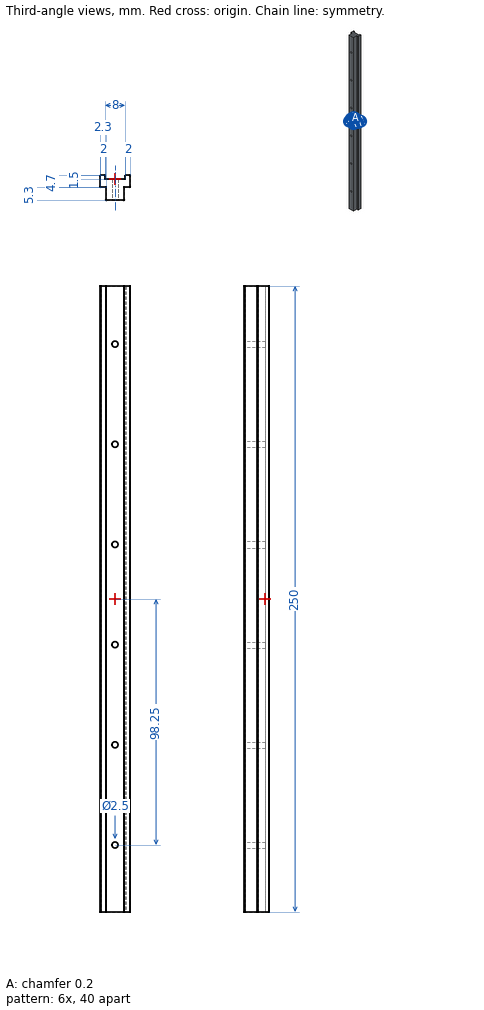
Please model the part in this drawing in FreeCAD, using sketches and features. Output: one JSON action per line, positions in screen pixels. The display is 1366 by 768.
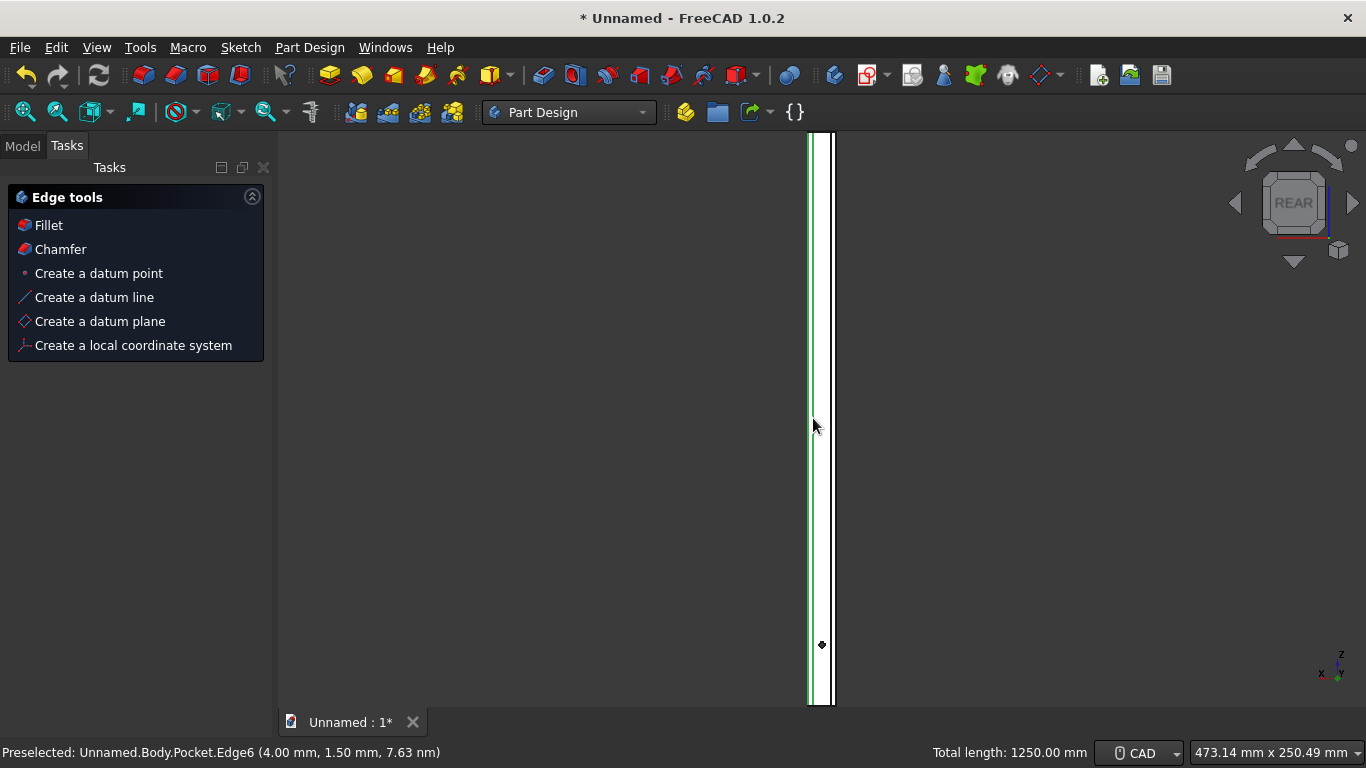
{"action": "left_click", "coordinate": [831, 418], "text": "ctrl"}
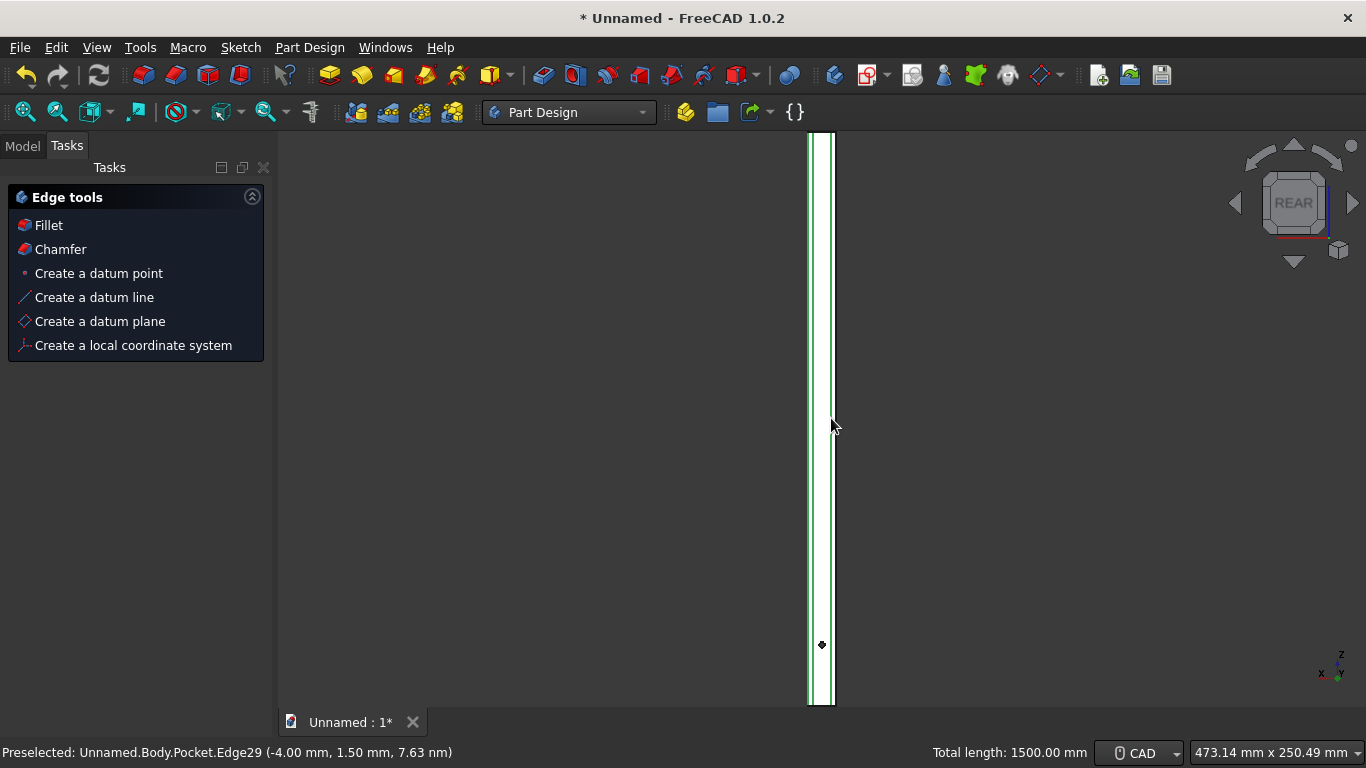
{"action": "key", "text": "6"}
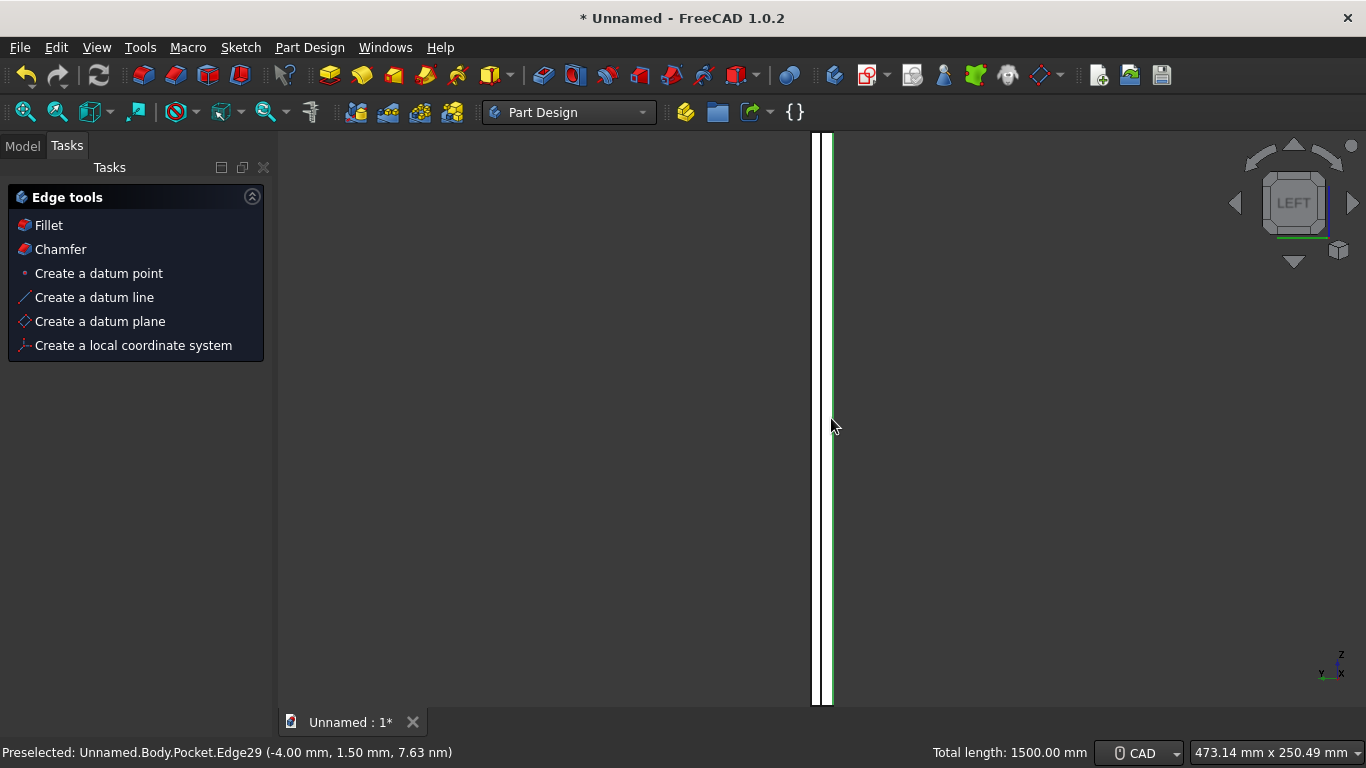
{"action": "left_click", "coordinate": [821, 418], "text": "ctrl"}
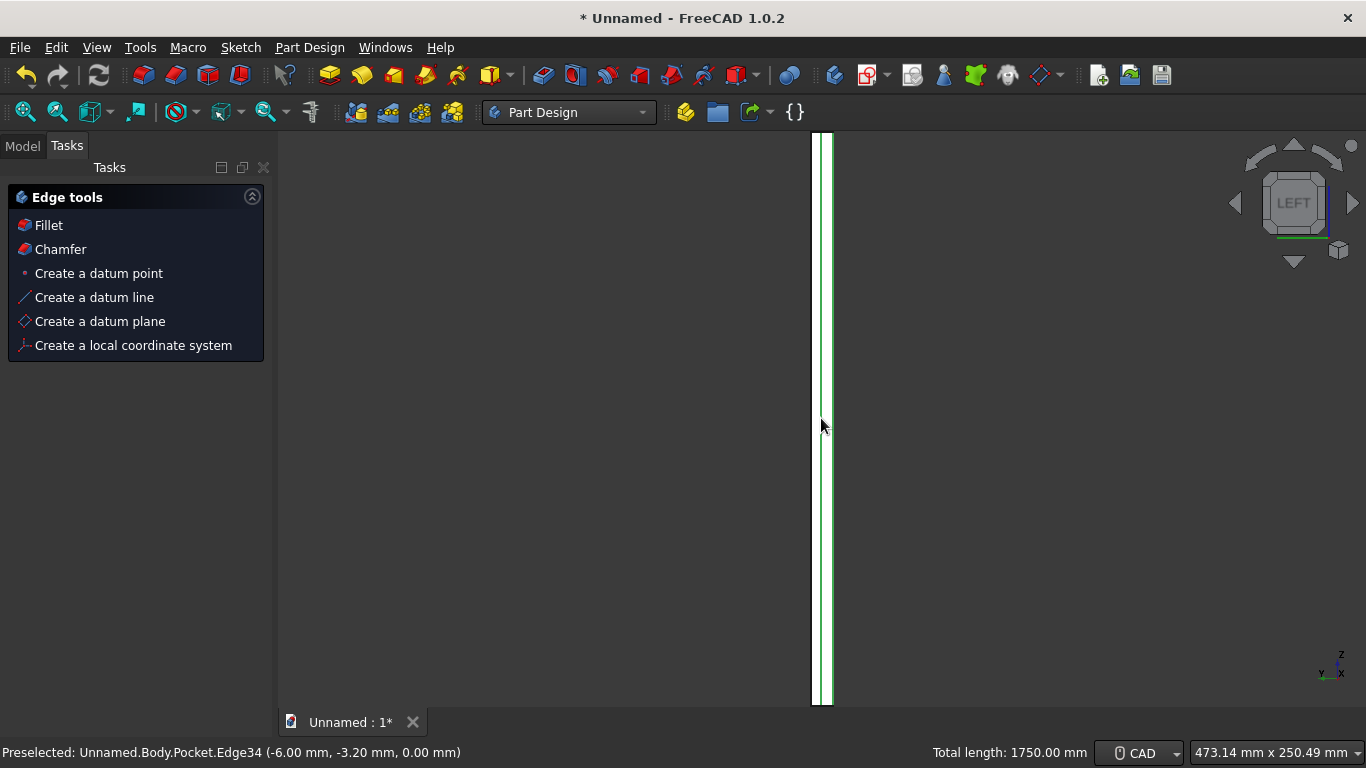
{"action": "left_click", "coordinate": [811, 418], "text": "ctrl"}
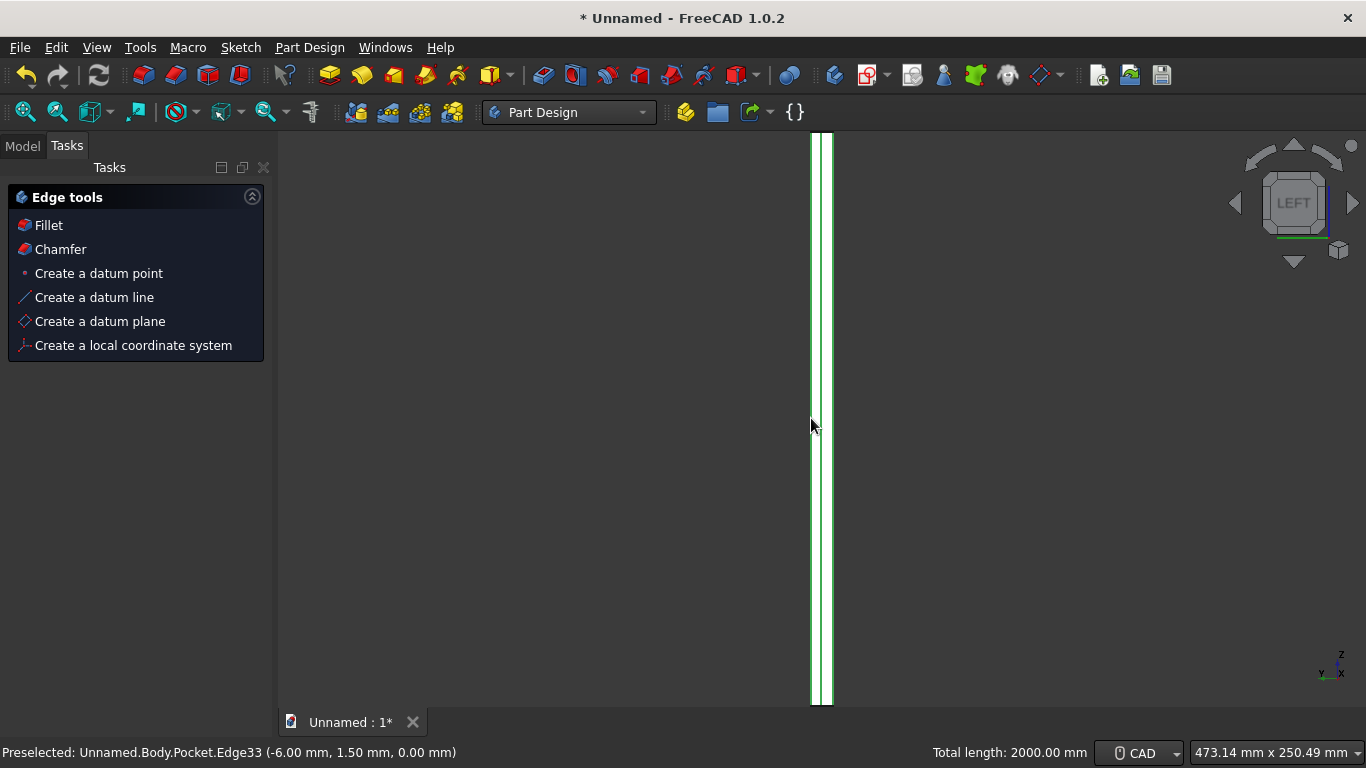
{"action": "left_click", "coordinate": [176, 76]}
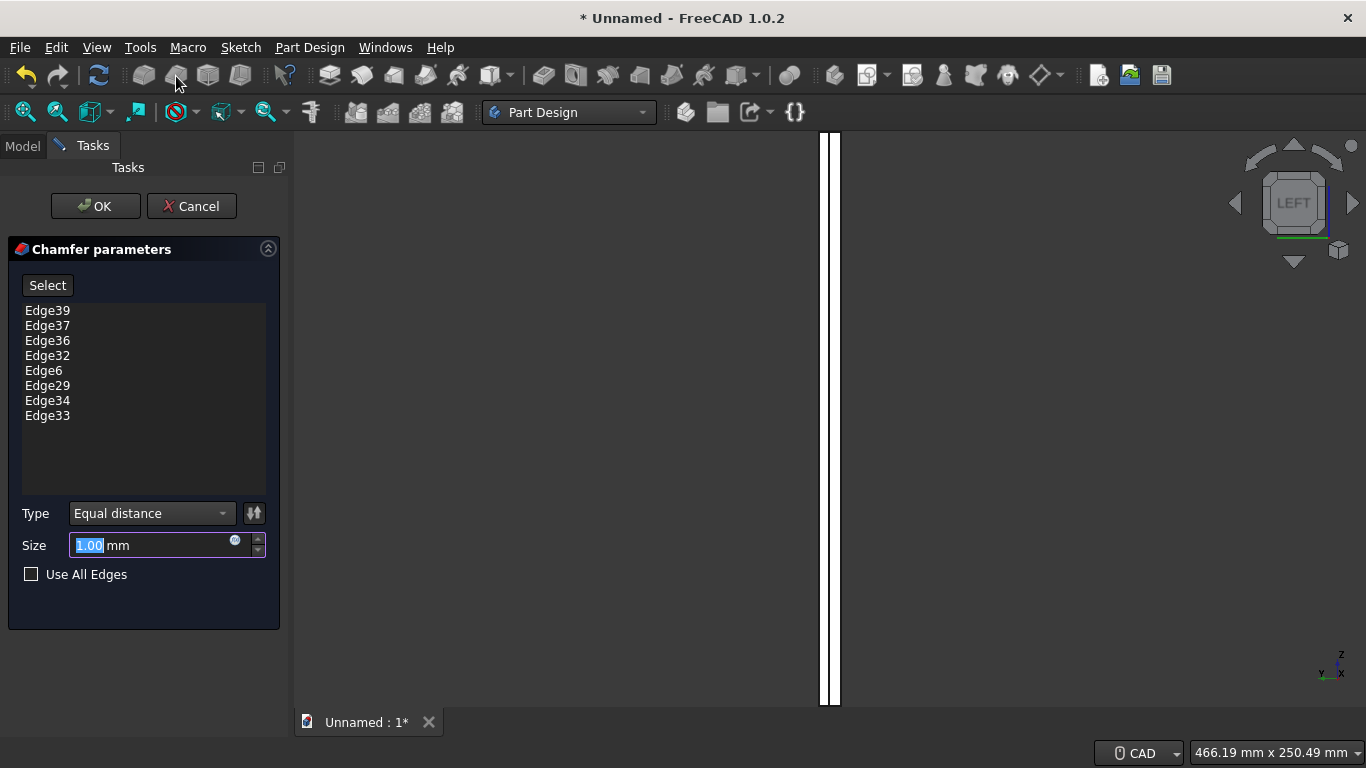
{"action": "type", "text": "0.2"}
{"action": "key", "text": "Tab"}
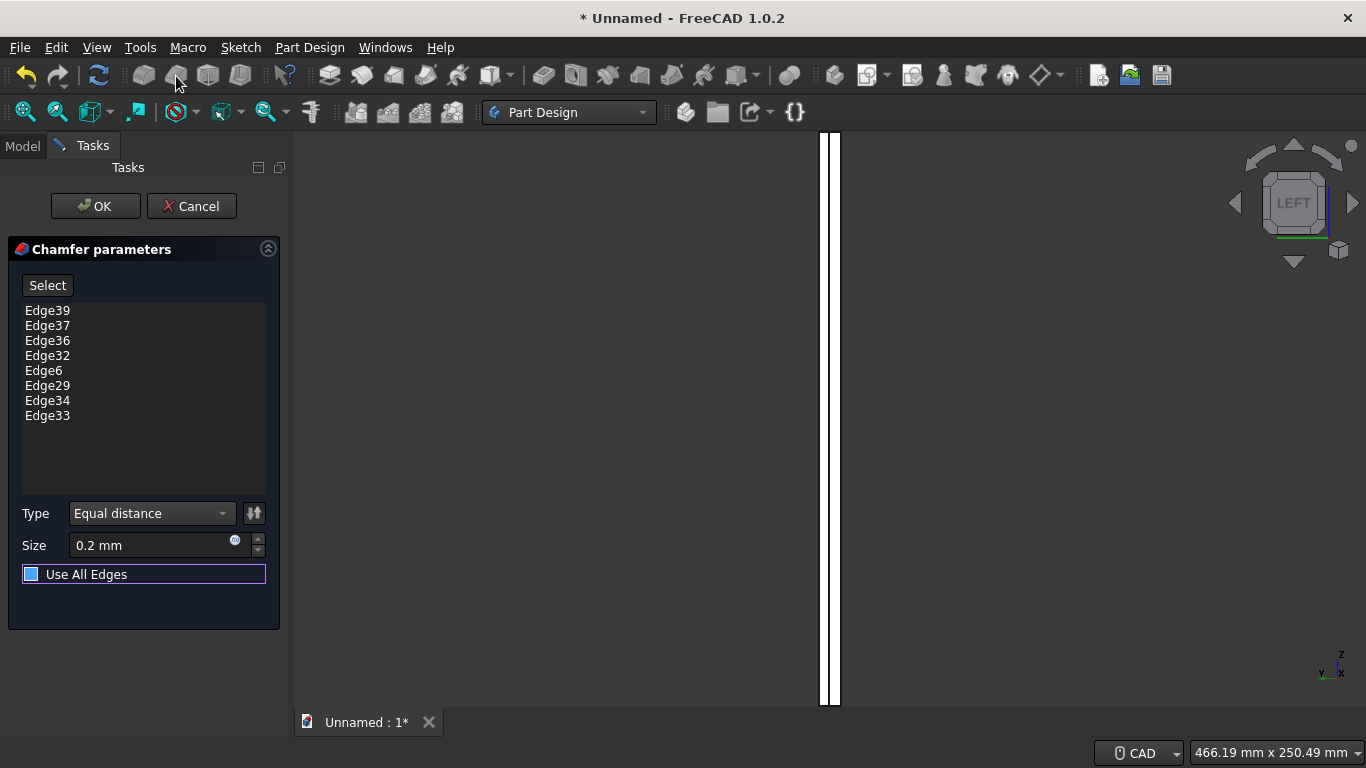
{"action": "left_click", "coordinate": [96, 206]}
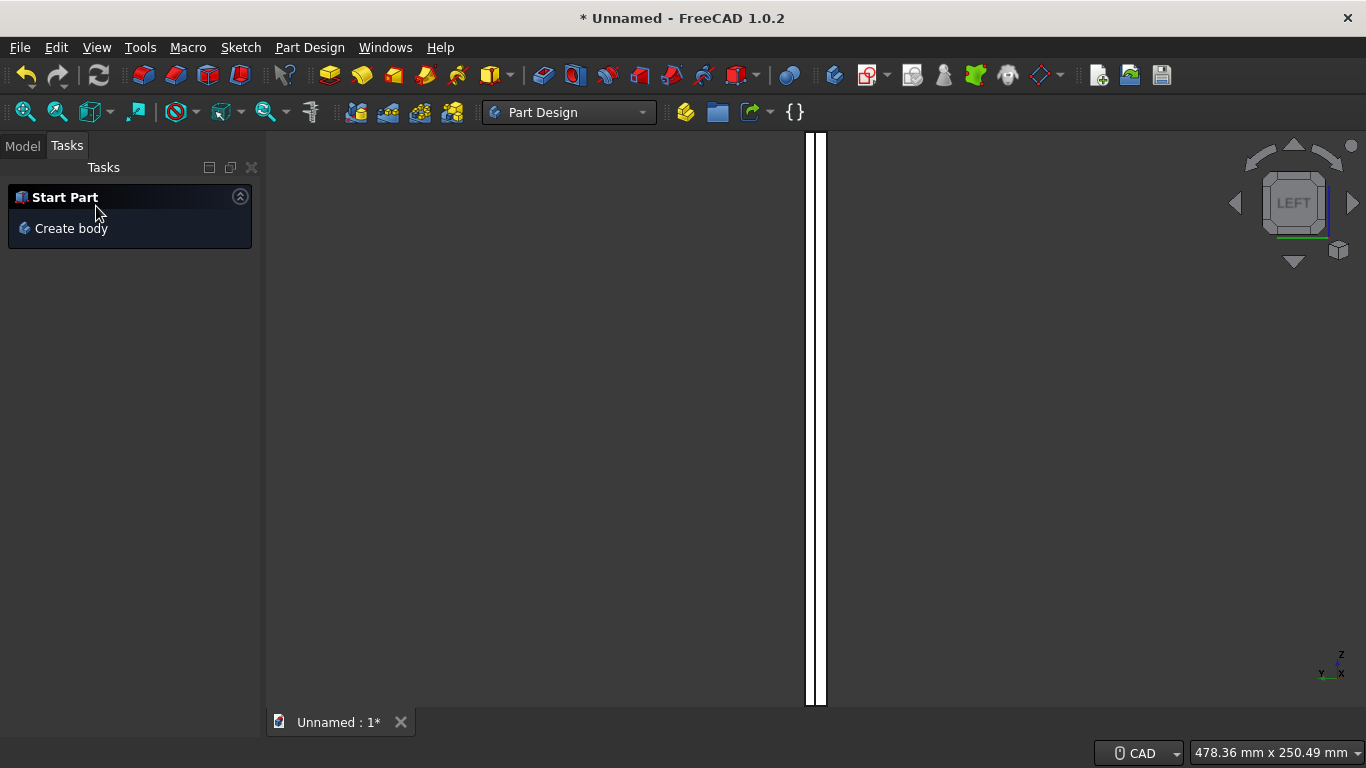
{"action": "left_click", "coordinate": [23, 145]}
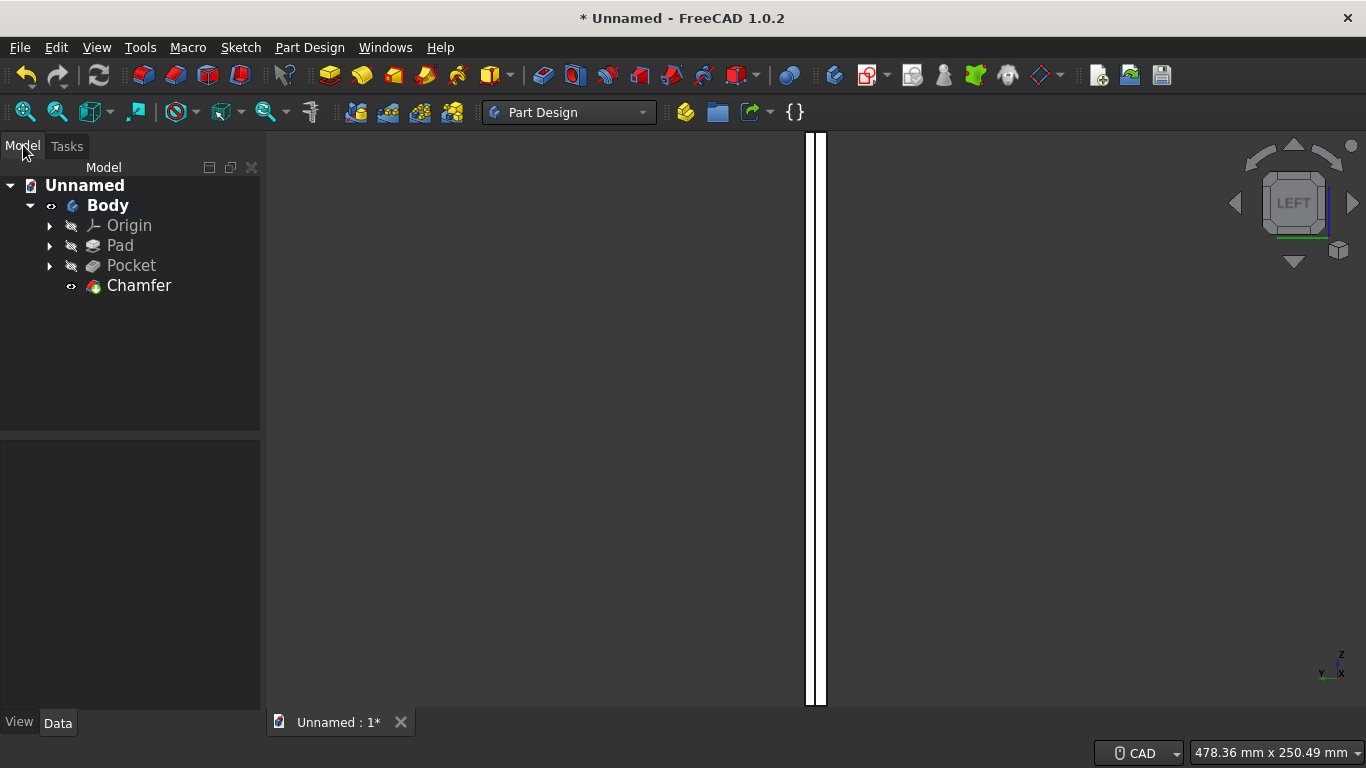
{"action": "left_click", "coordinate": [116, 266]}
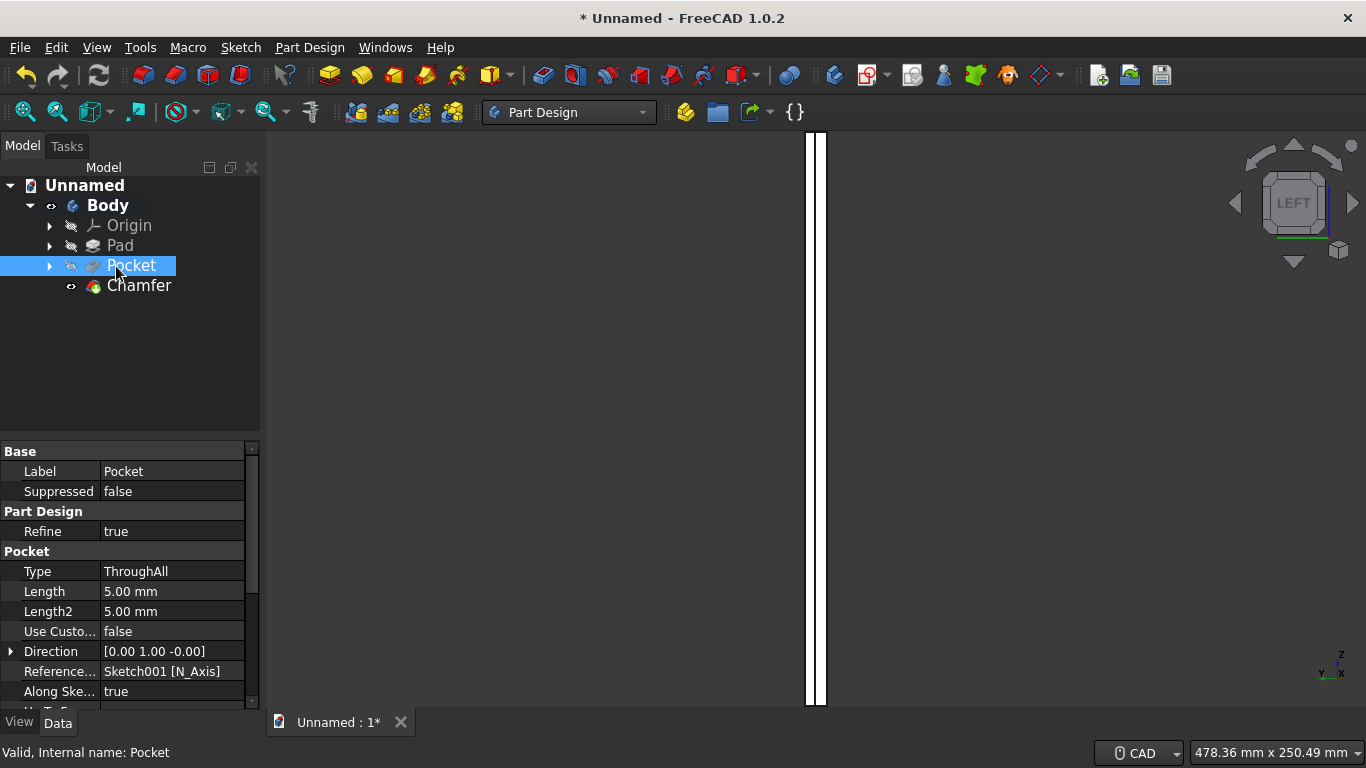
{"action": "left_click", "coordinate": [388, 112]}